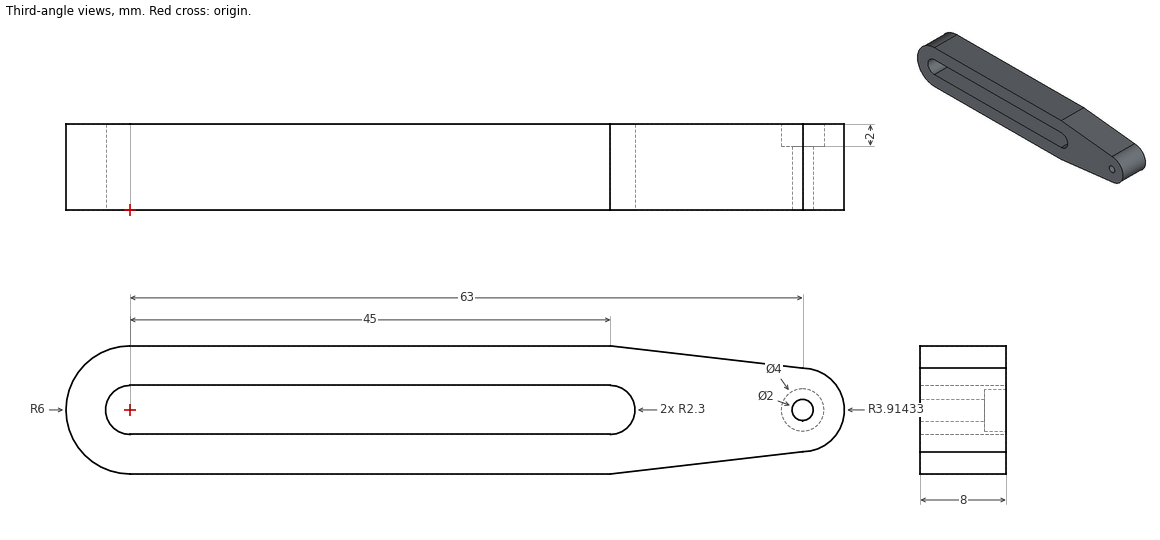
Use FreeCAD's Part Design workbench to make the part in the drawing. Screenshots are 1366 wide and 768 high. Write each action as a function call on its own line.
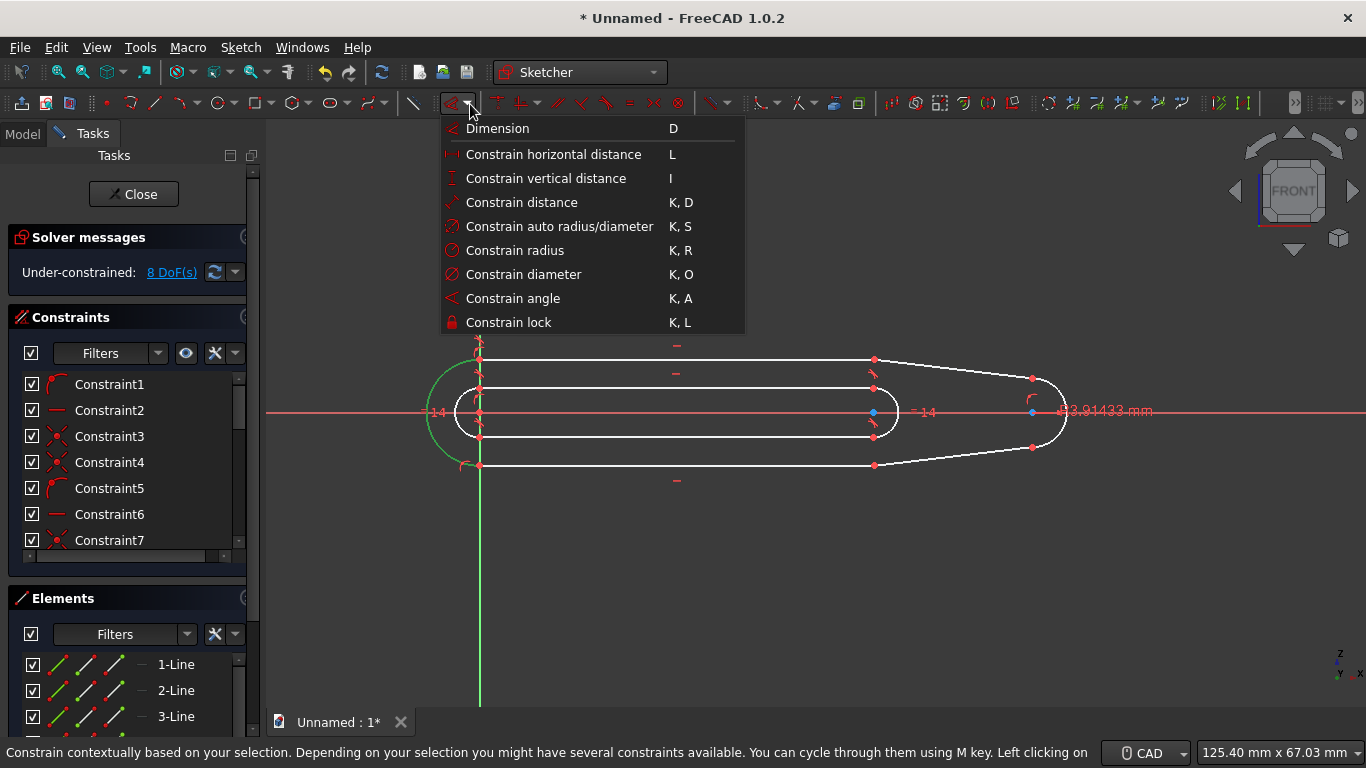
click(593, 250)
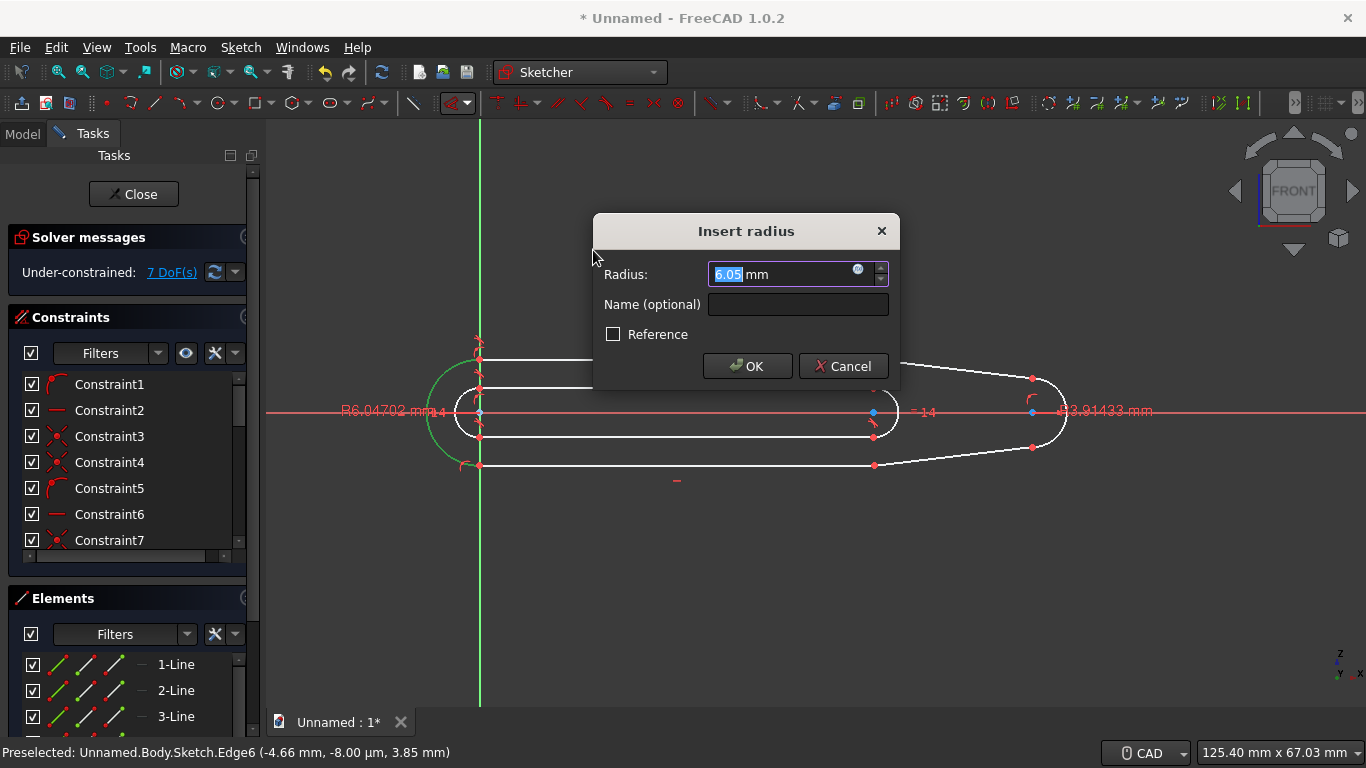
text(6)
key(Return)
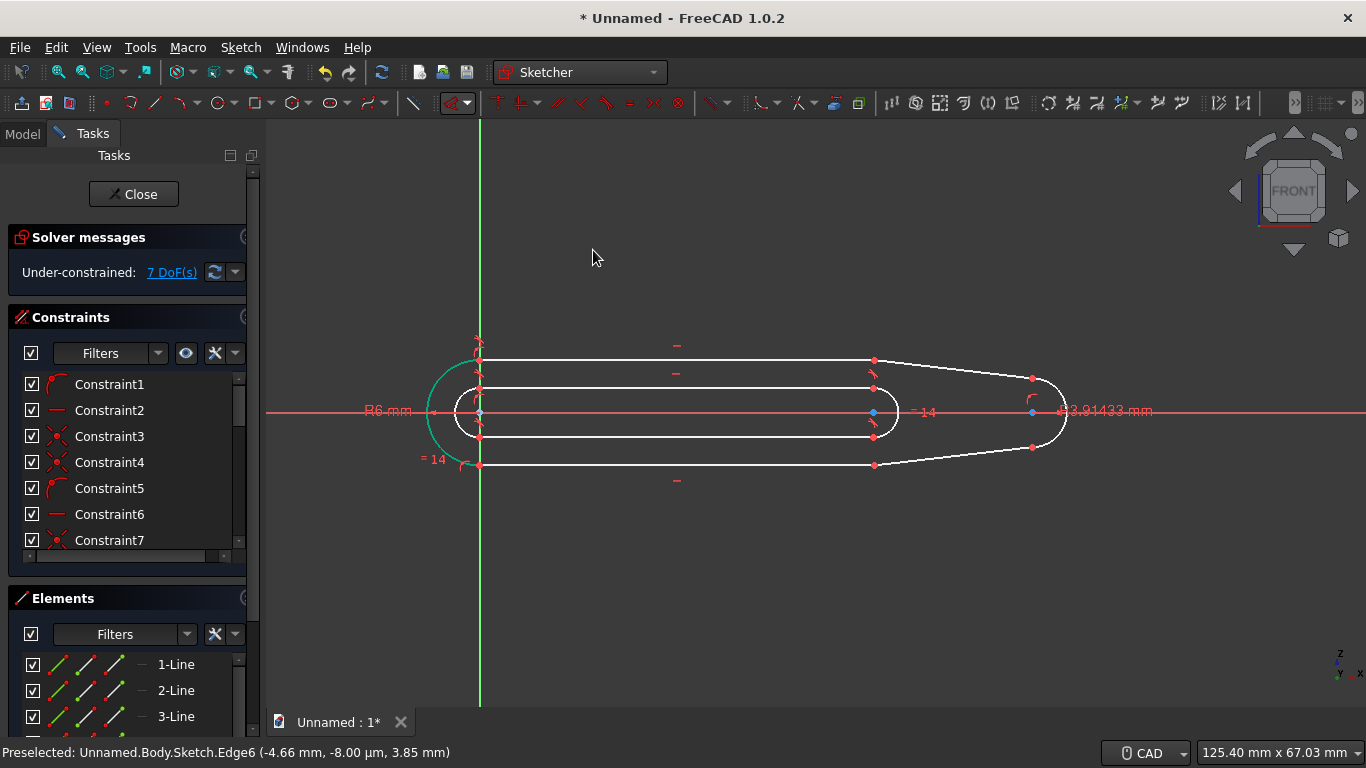
scroll(460, 398, up, 4)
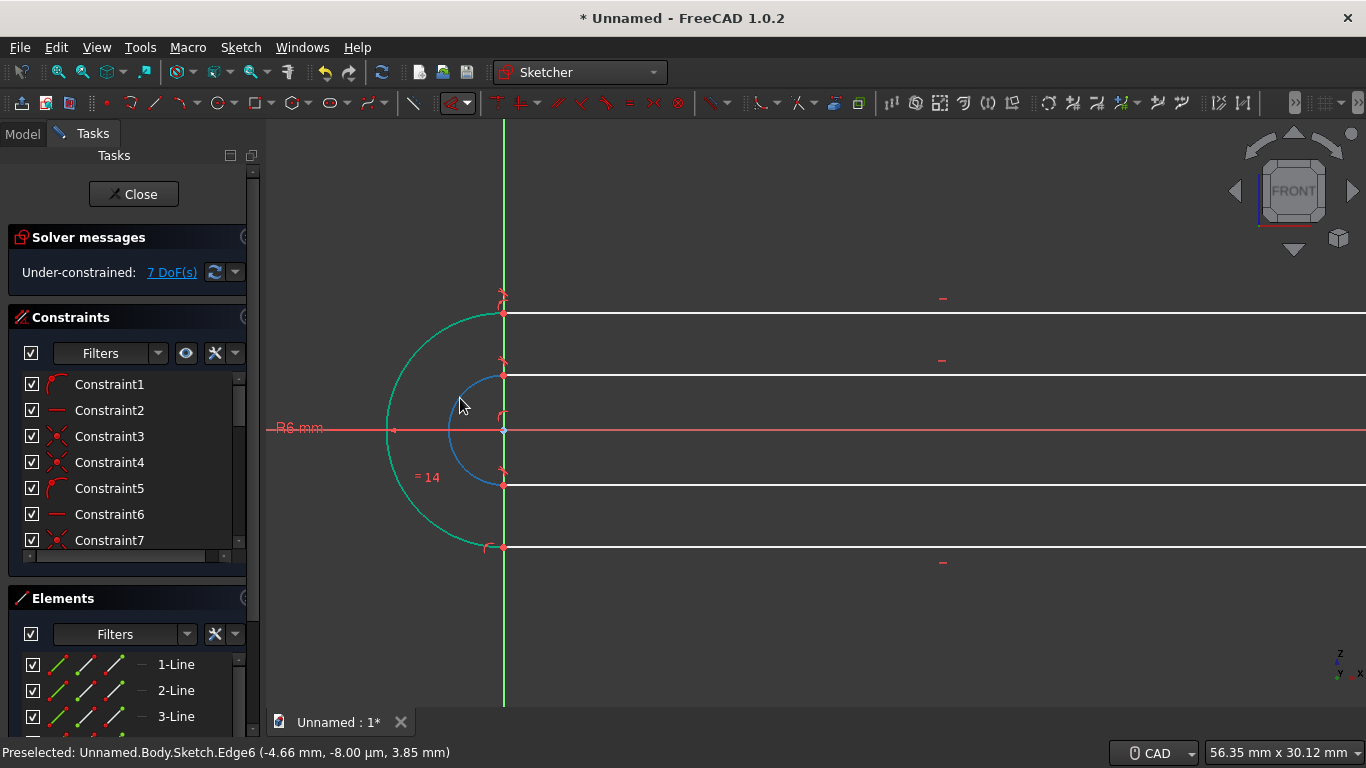
click(459, 398)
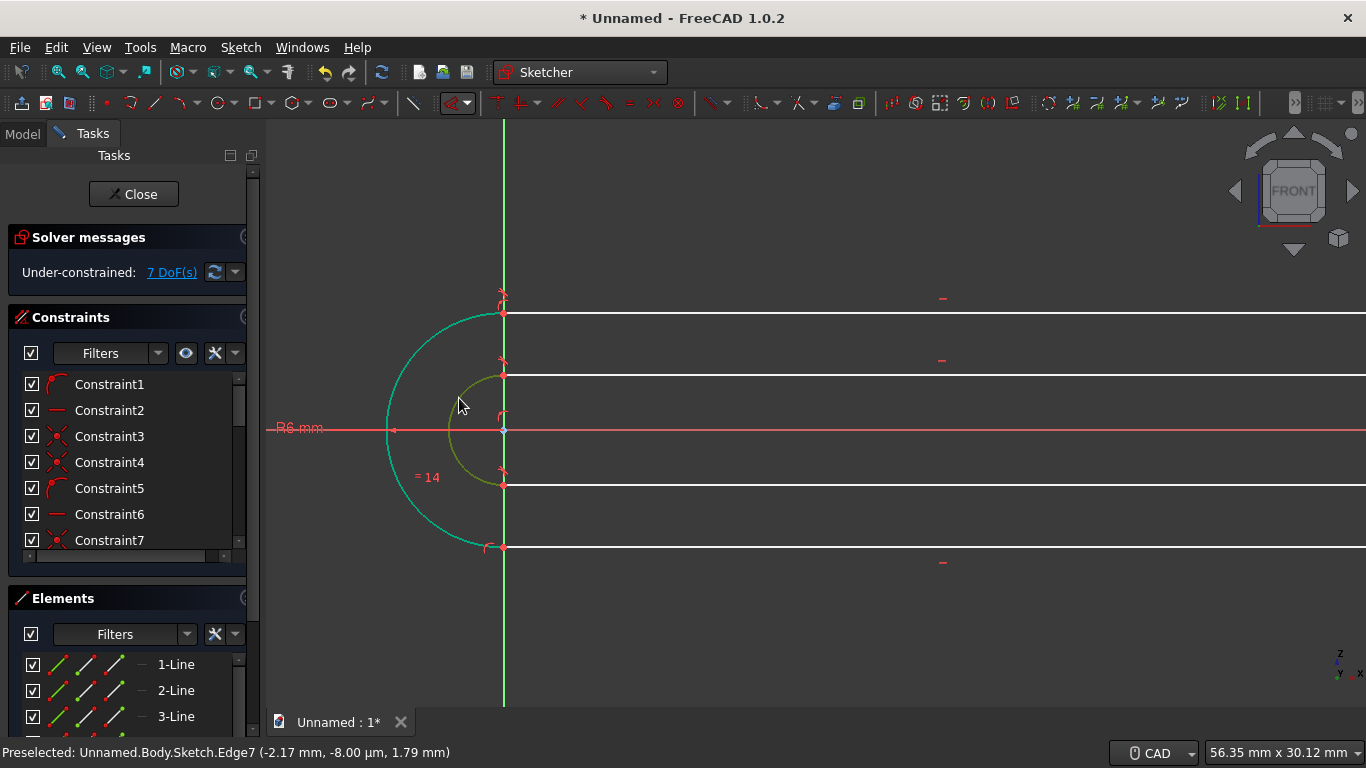
key(k)
key(r)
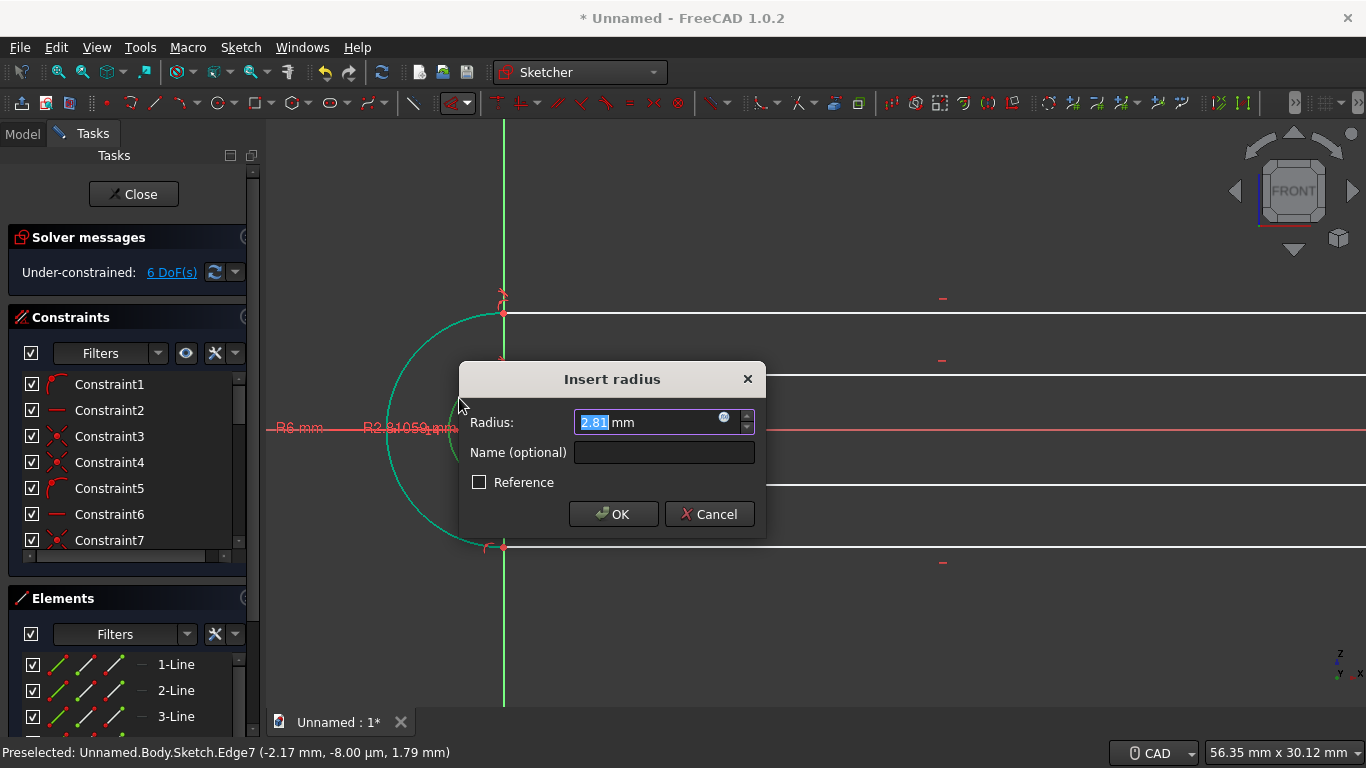
text(2.3)
key(Return)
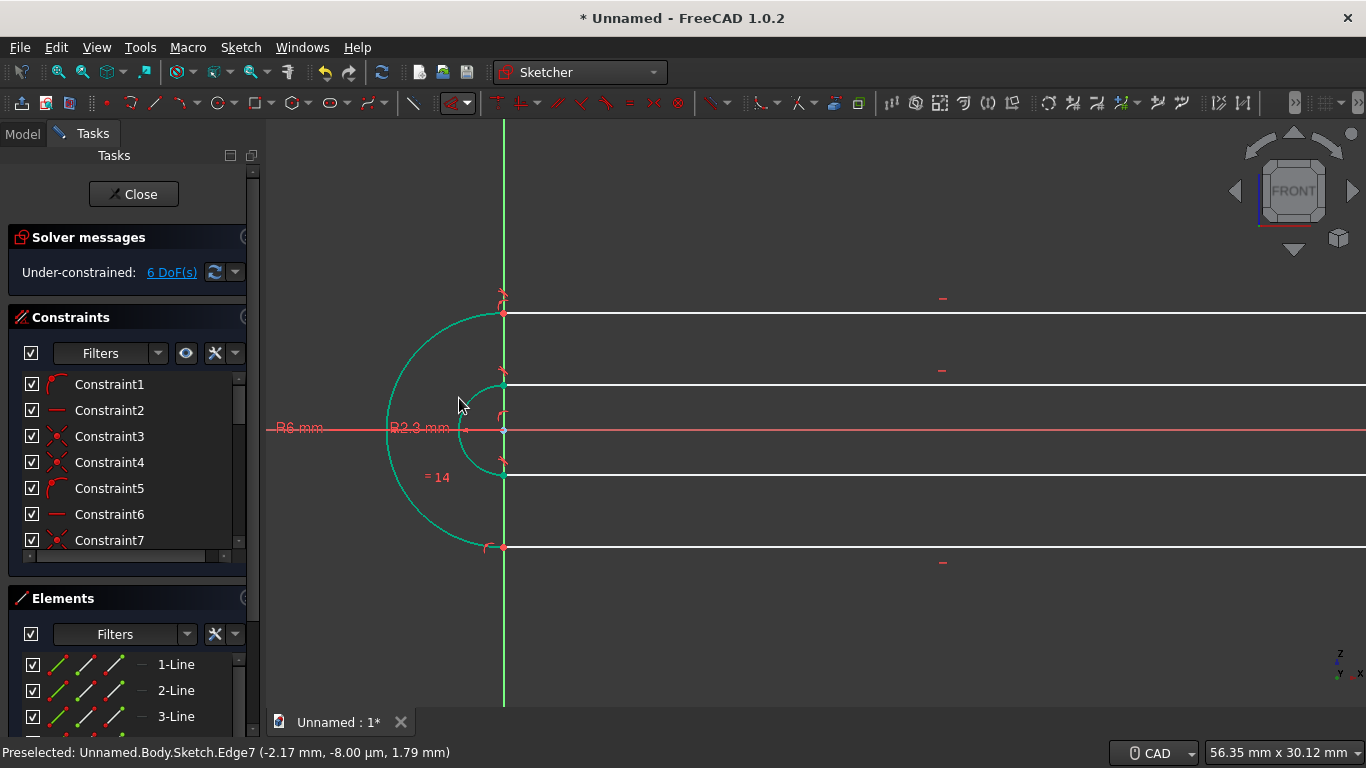
click(768, 313)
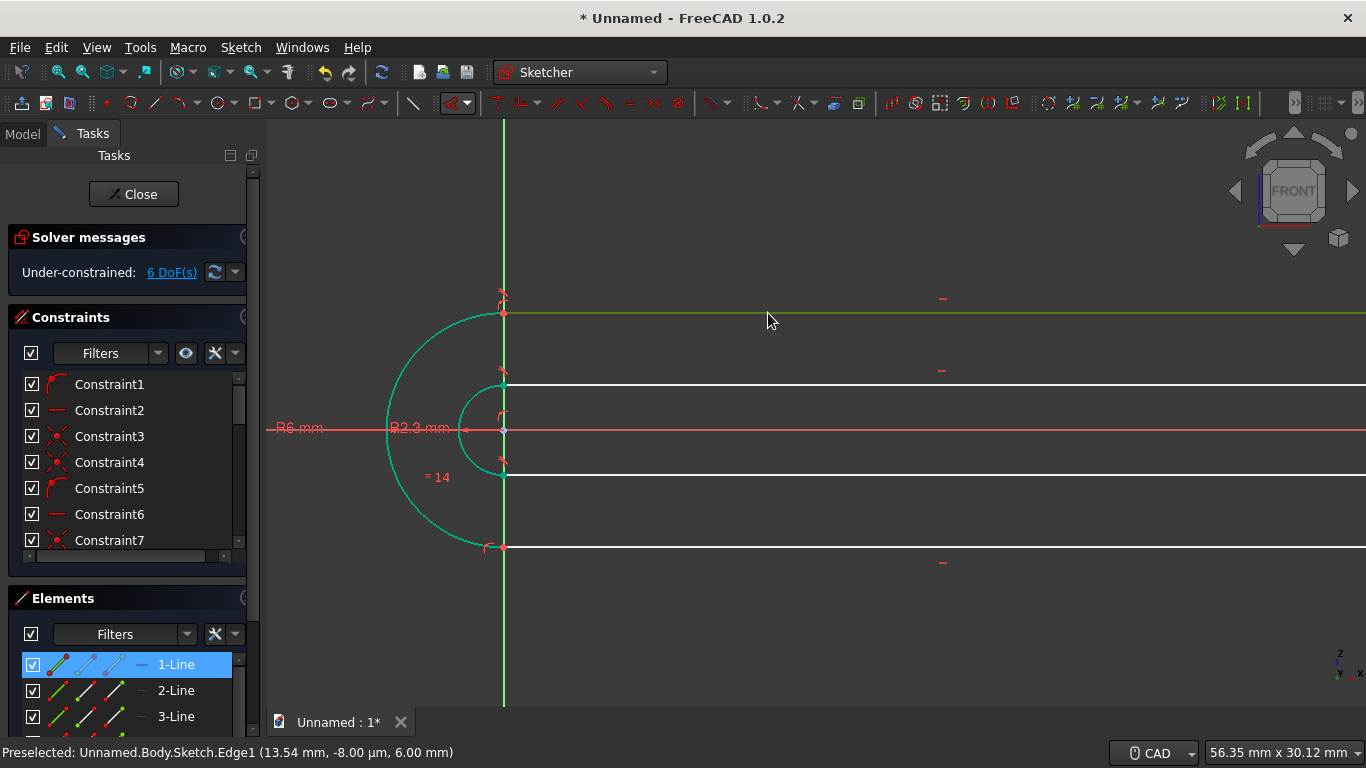
click(470, 104)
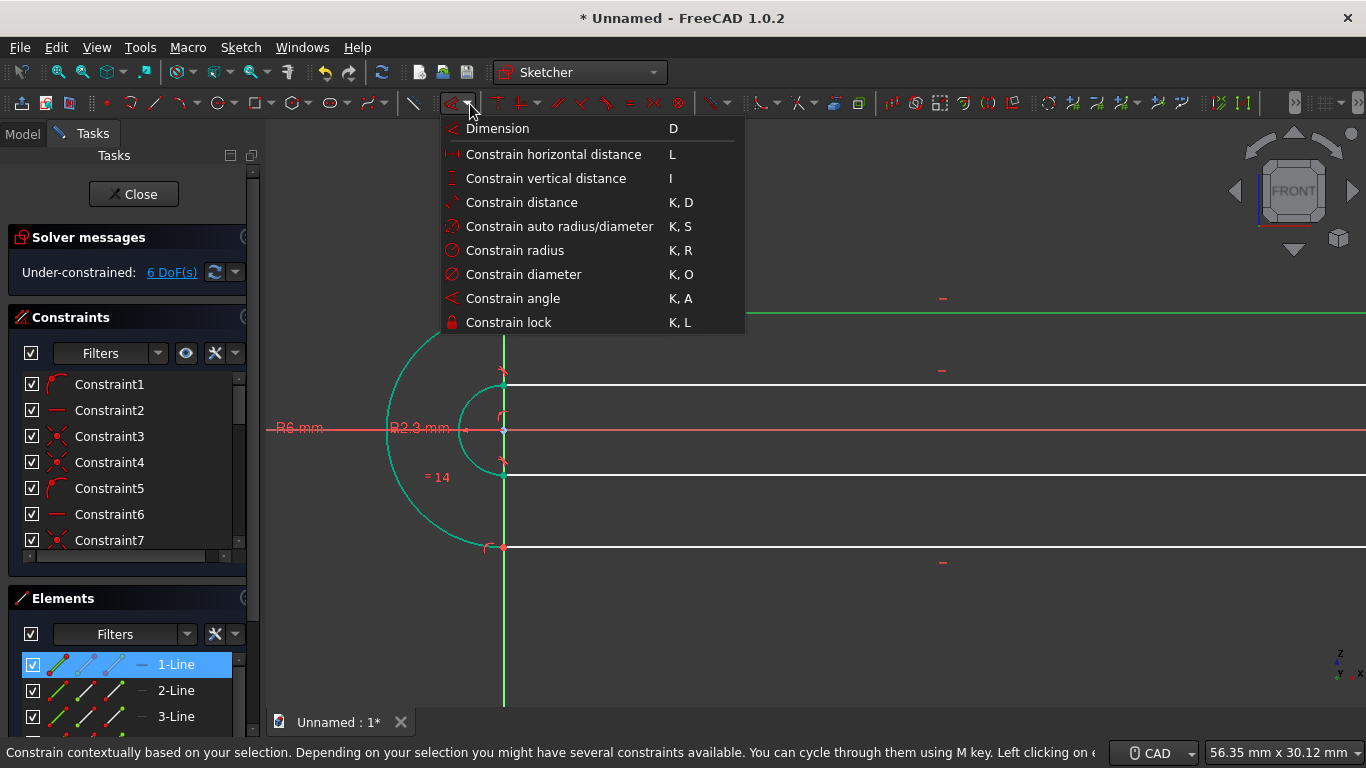
click(593, 154)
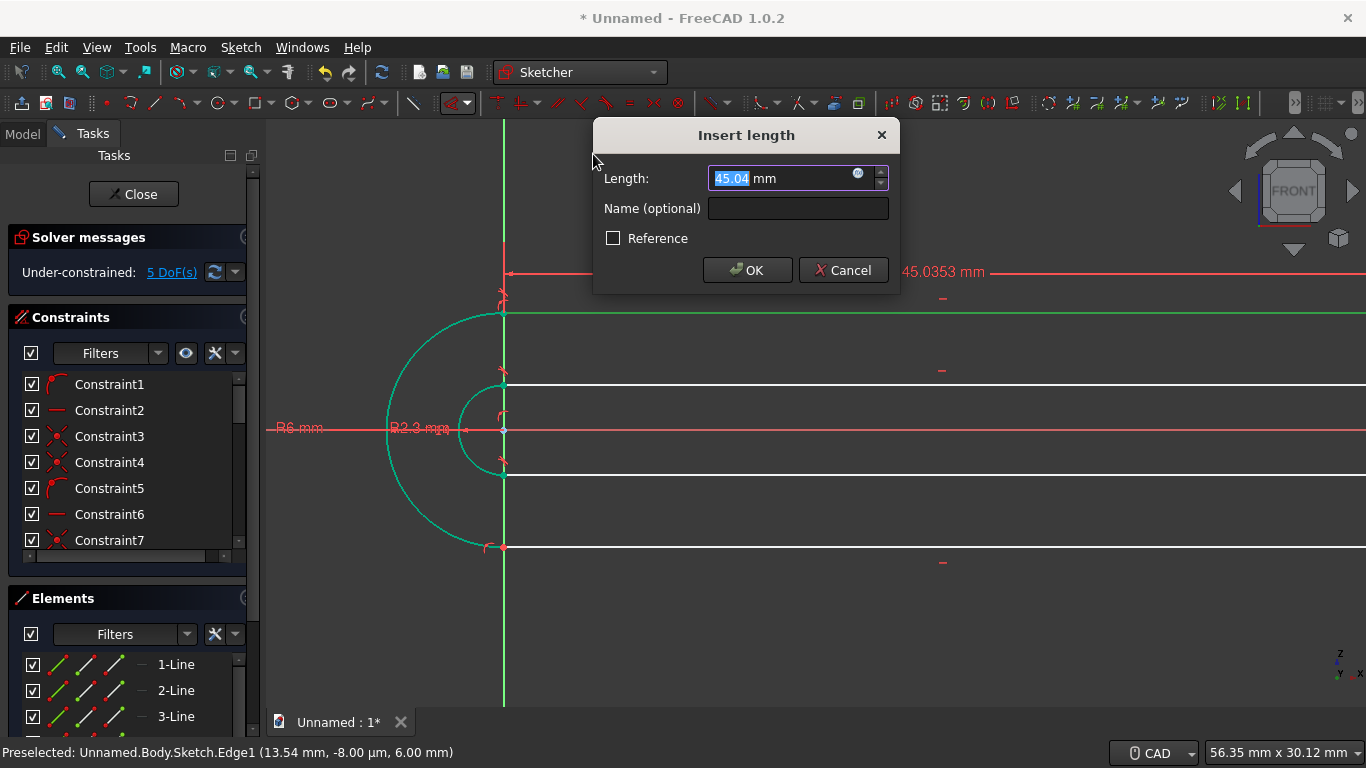
text(45)
key(Return)